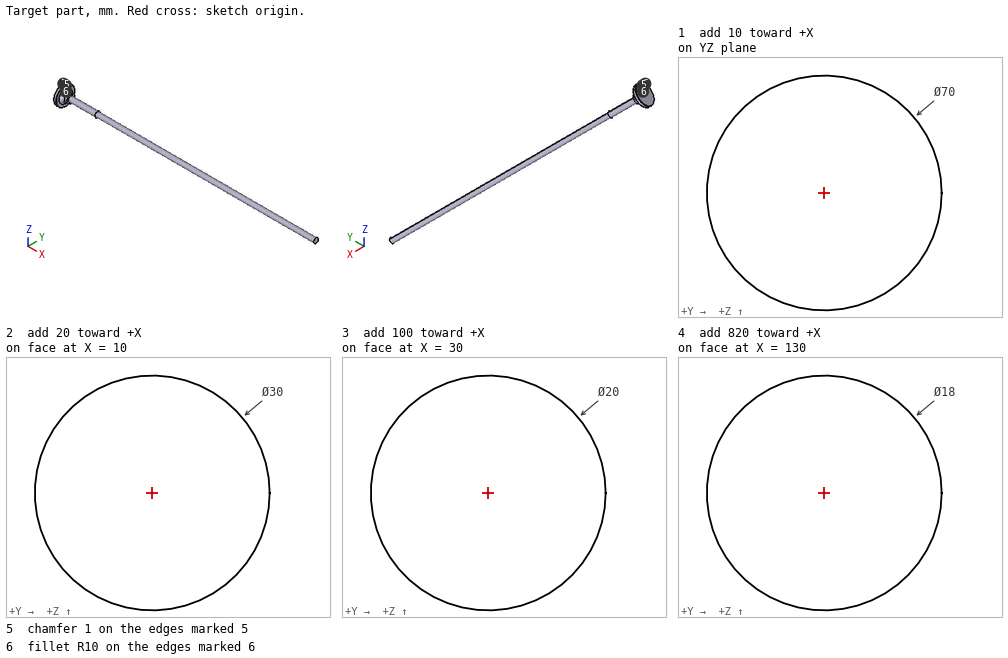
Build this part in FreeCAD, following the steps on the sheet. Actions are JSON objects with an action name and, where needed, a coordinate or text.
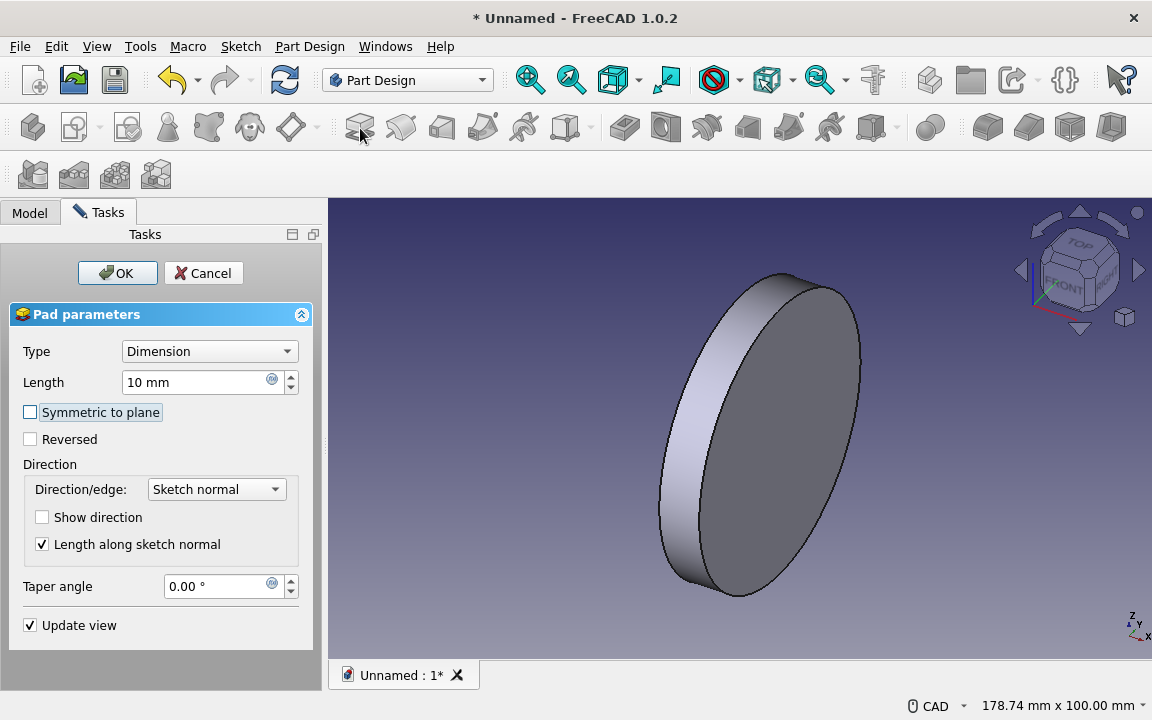
{"action": "left_click", "coordinate": [118, 273]}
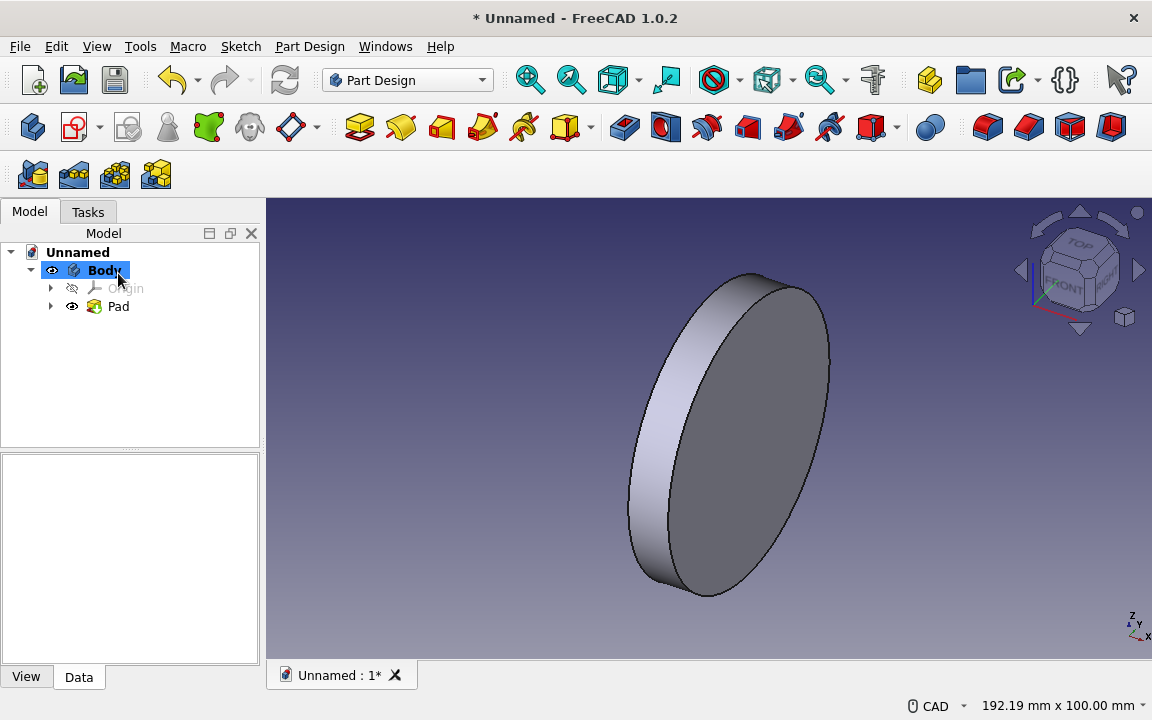
{"action": "left_click", "coordinate": [749, 441]}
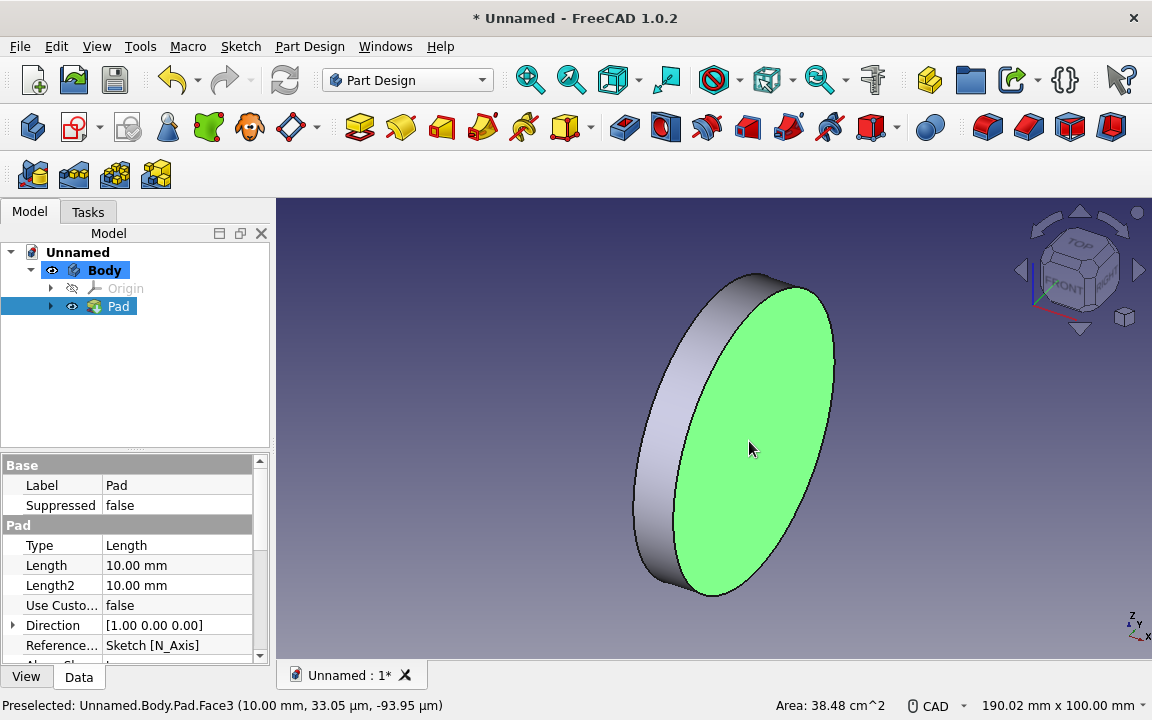
{"action": "left_click", "coordinate": [74, 128]}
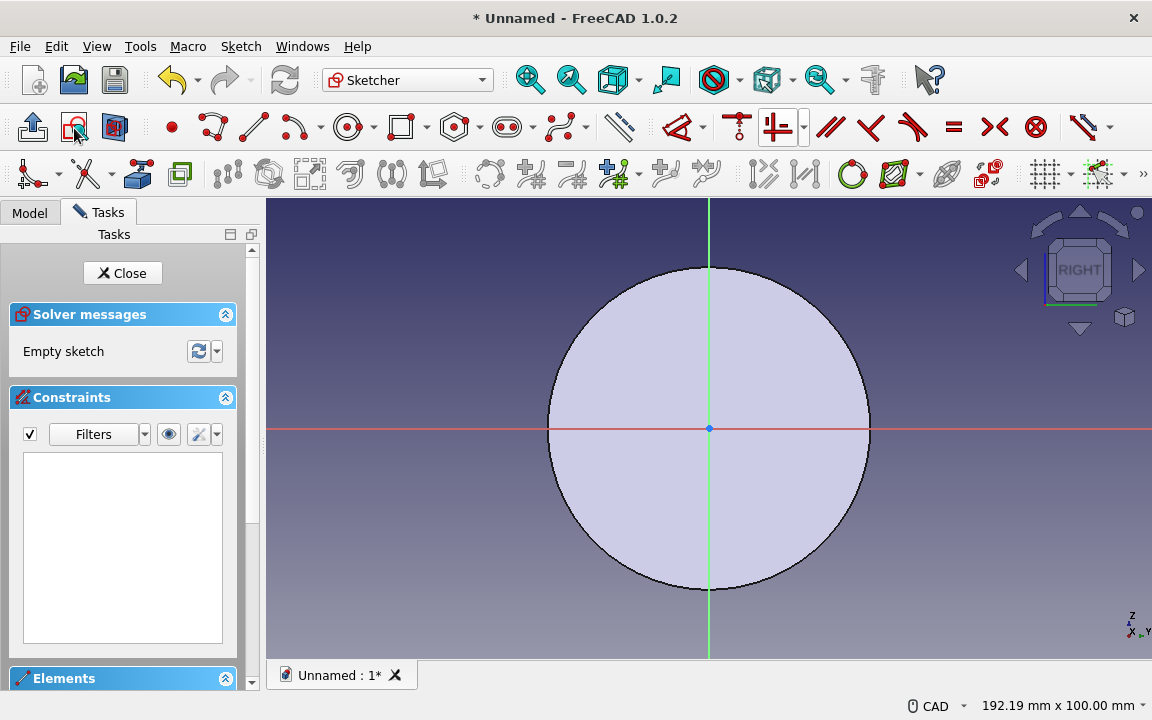
{"action": "scroll", "coordinate": [765, 428], "scroll_direction": "up", "scroll_amount": 4}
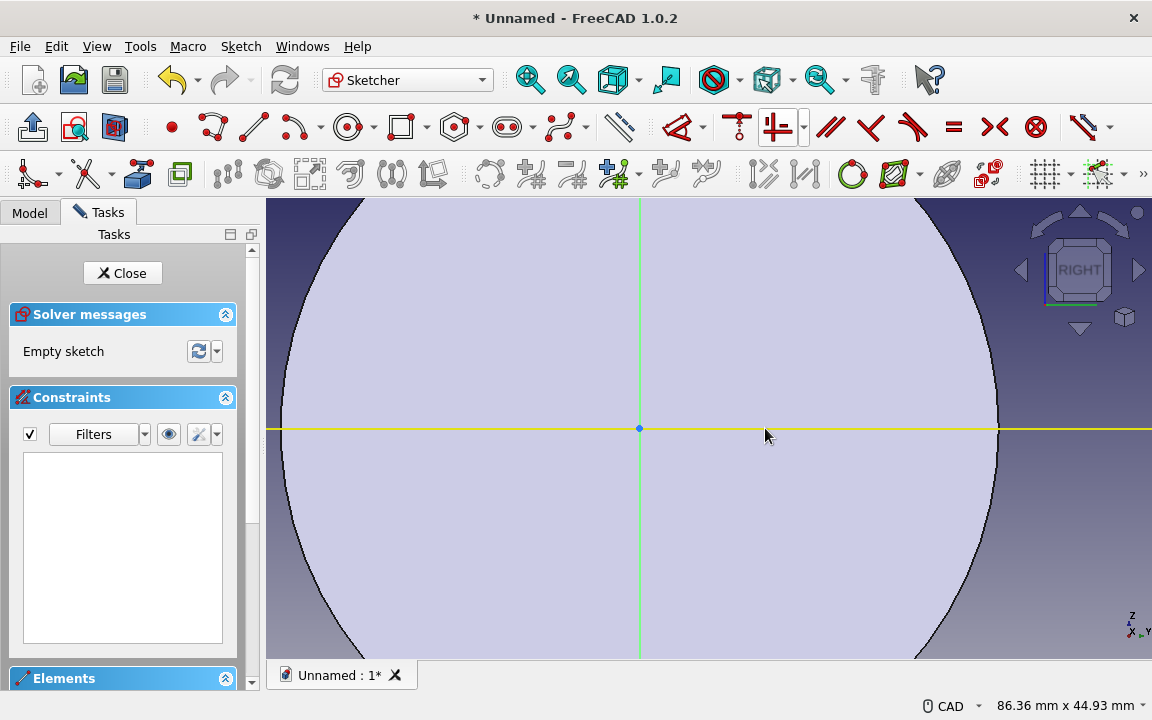
{"action": "left_click", "coordinate": [348, 128]}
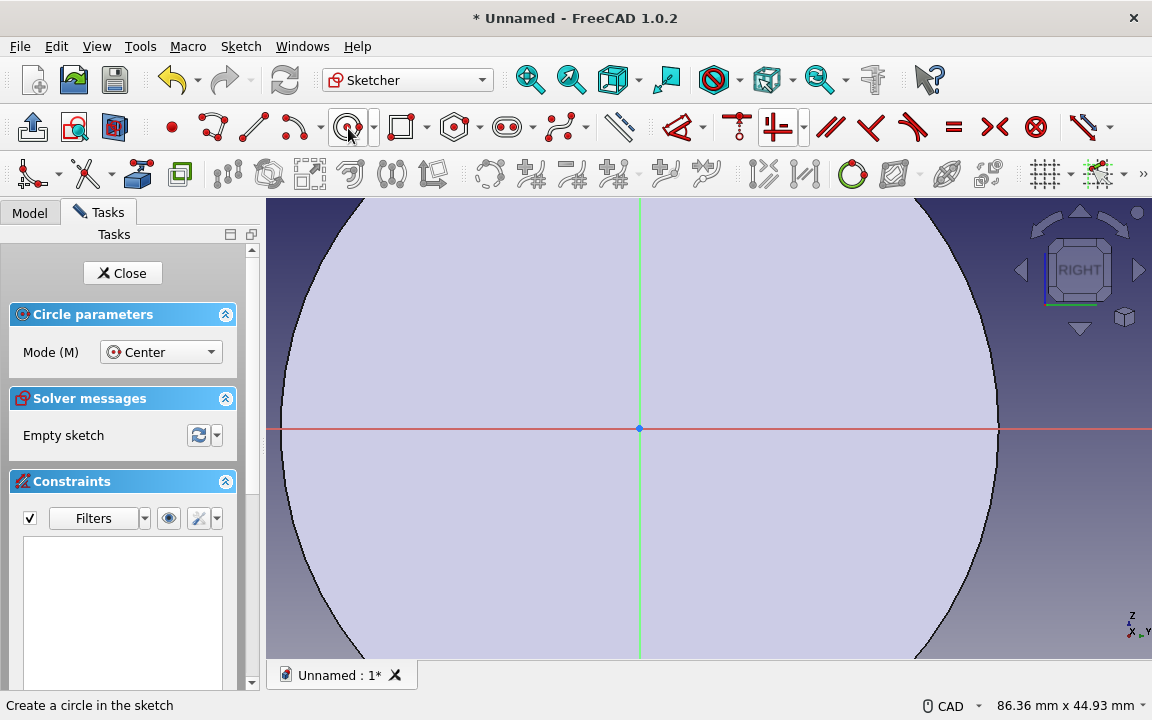
{"action": "left_click", "coordinate": [640, 428]}
{"action": "left_click", "coordinate": [748, 320]}
{"action": "key", "text": "Escape"}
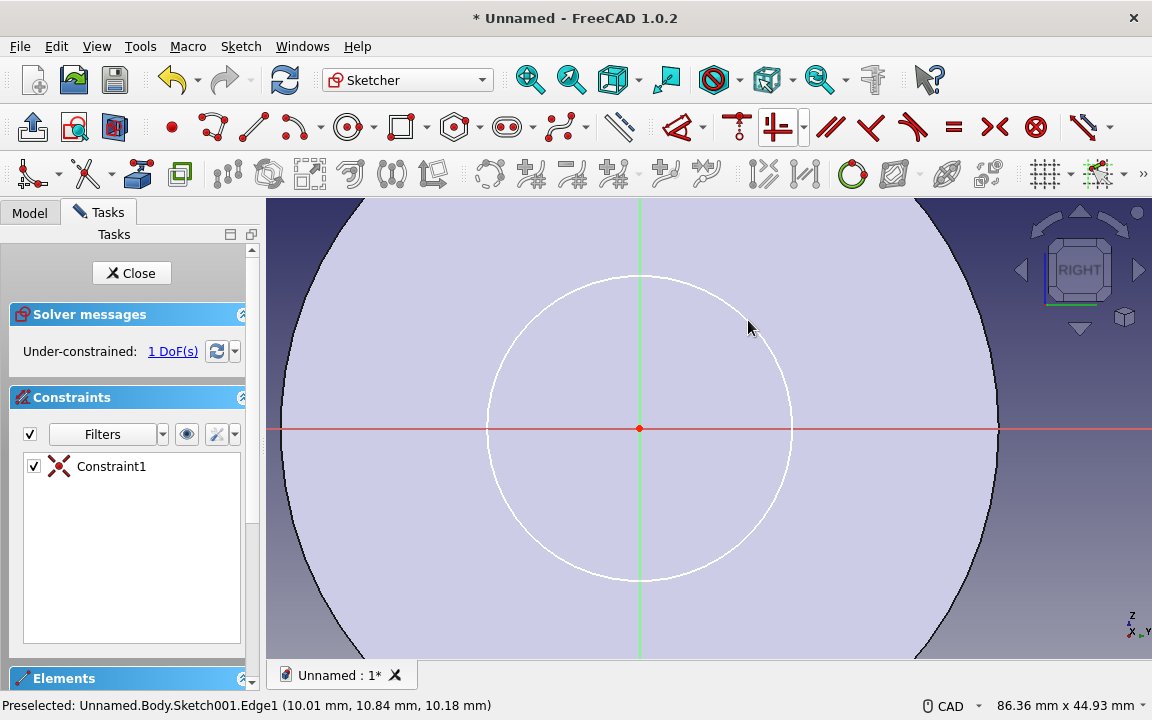
{"action": "key", "text": "d"}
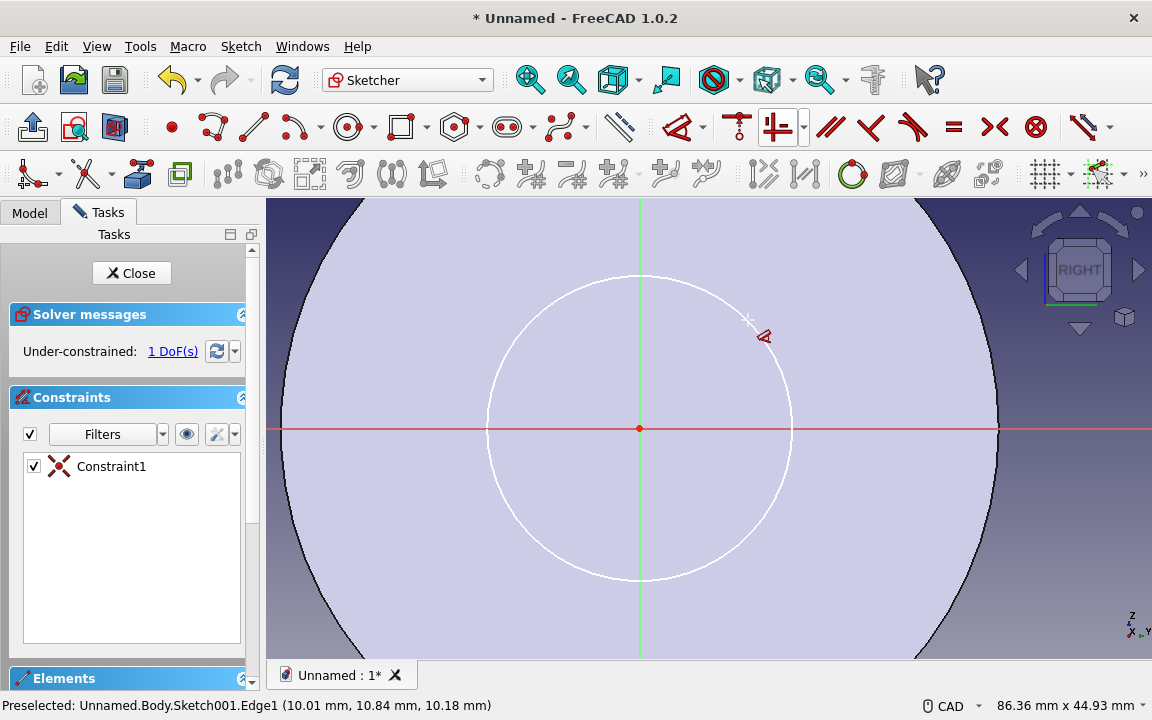
{"action": "left_click", "coordinate": [747, 320]}
{"action": "left_click", "coordinate": [770, 297]}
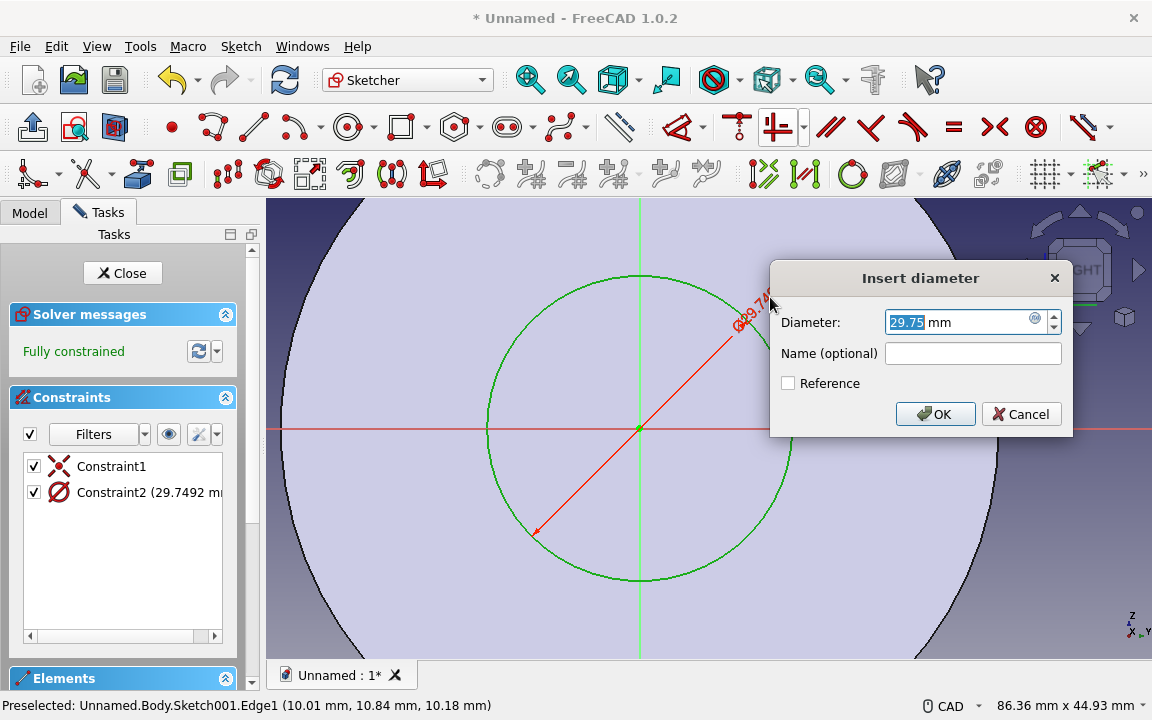
{"action": "type", "text": "30"}
{"action": "key", "text": "Return"}
{"action": "key", "text": "Escape"}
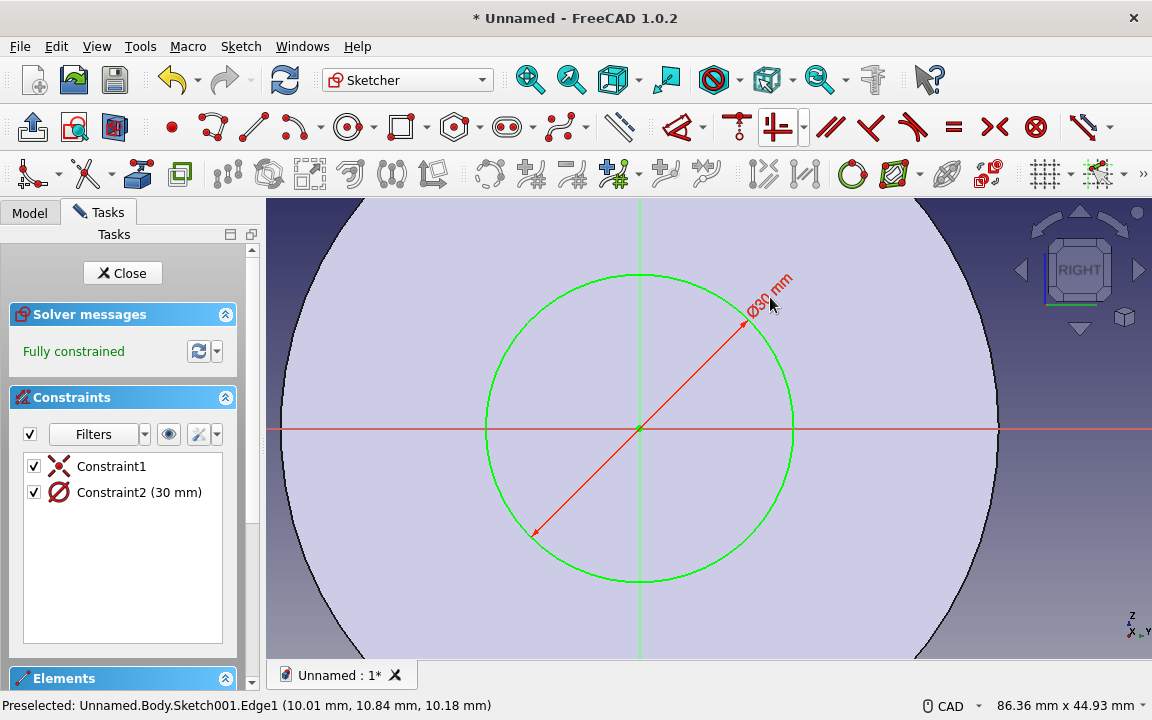
{"action": "left_click", "coordinate": [123, 273]}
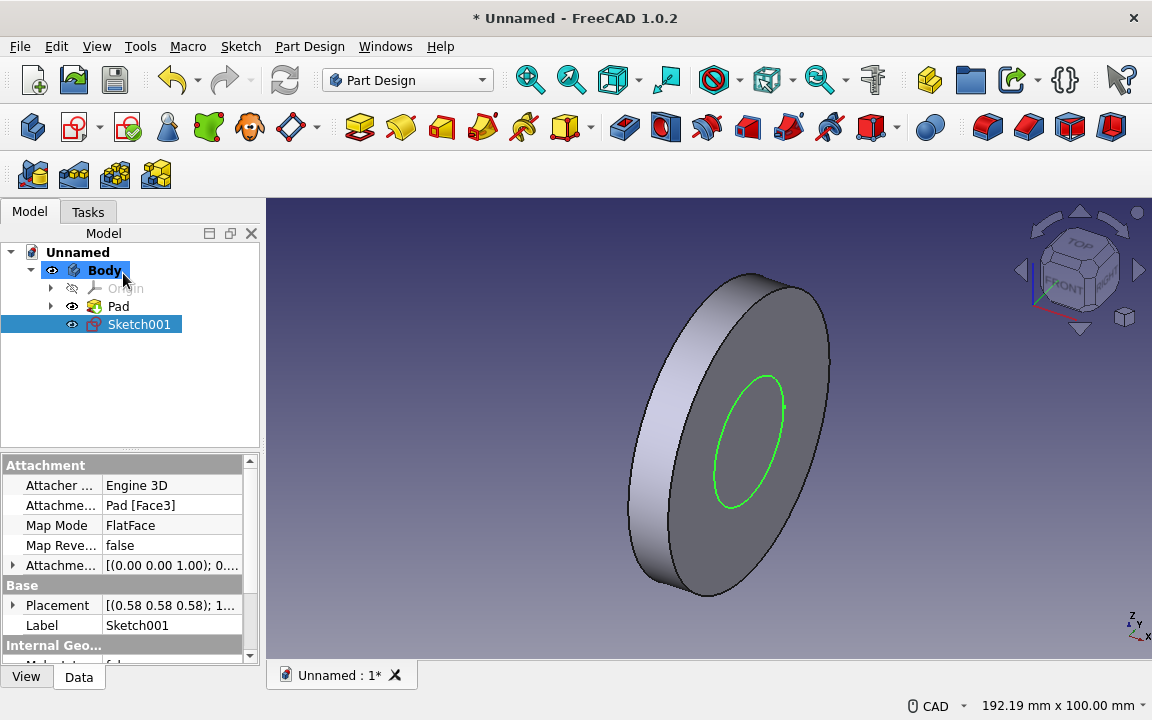
{"action": "left_click", "coordinate": [360, 128]}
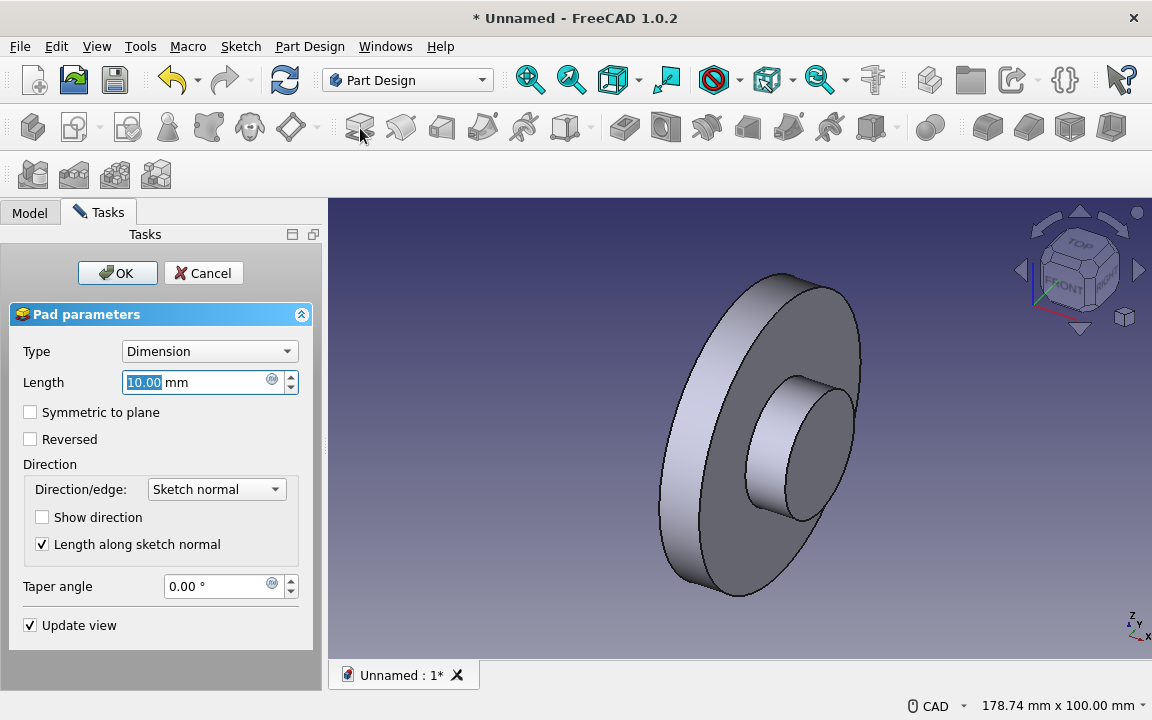
{"action": "type", "text": "20"}
{"action": "key", "text": "Tab"}